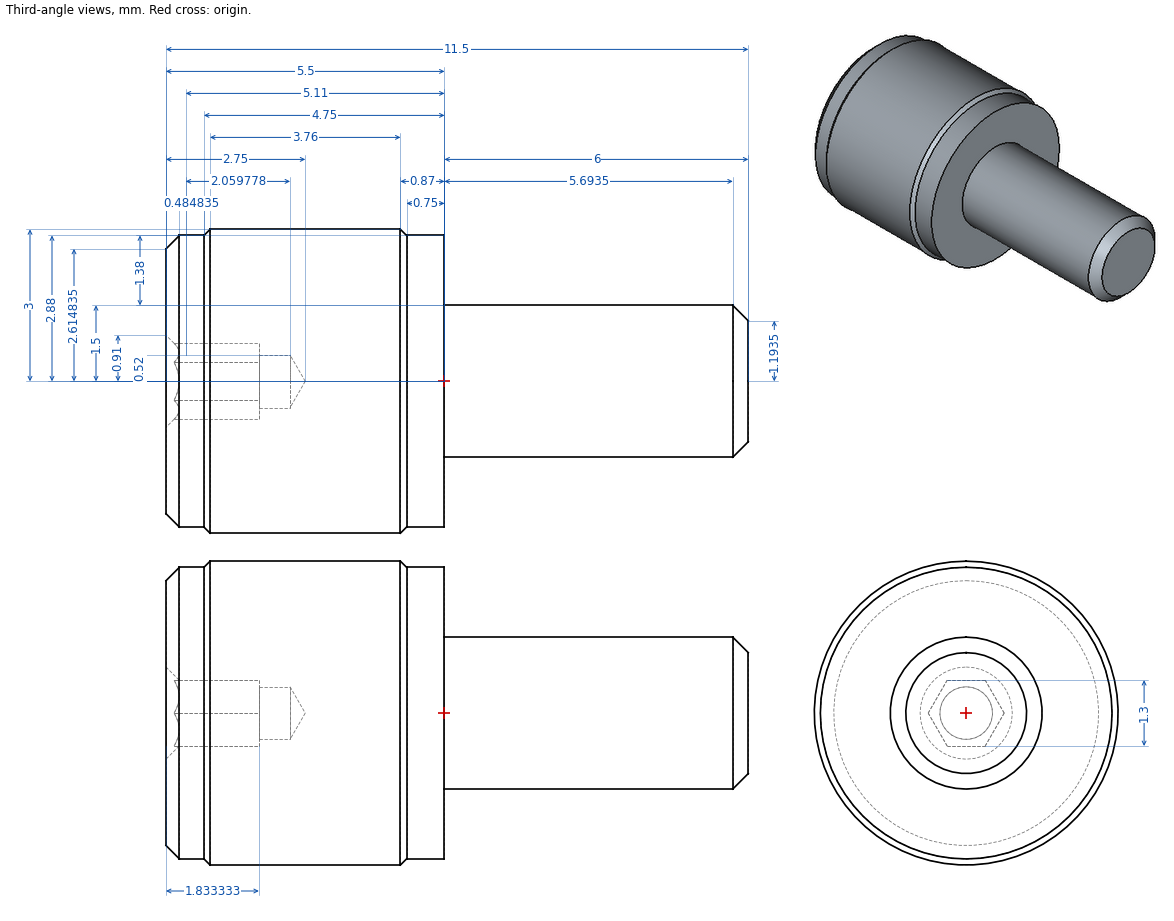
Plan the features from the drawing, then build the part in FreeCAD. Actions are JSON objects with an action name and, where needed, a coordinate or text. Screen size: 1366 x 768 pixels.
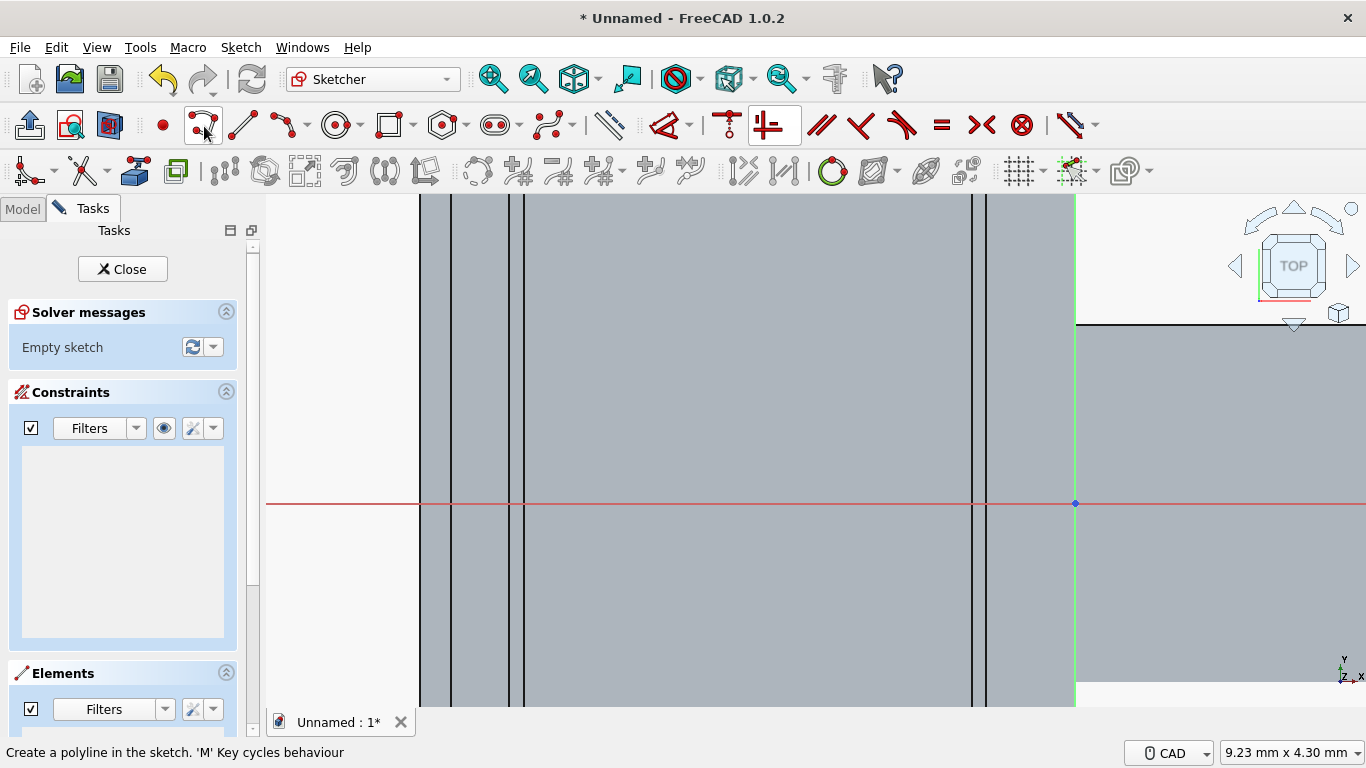
{"action": "left_click", "coordinate": [748, 504]}
{"action": "left_click", "coordinate": [712, 442]}
{"action": "left_click", "coordinate": [466, 442]}
{"action": "left_click", "coordinate": [420, 396]}
{"action": "left_click", "coordinate": [420, 495]}
{"action": "left_click", "coordinate": [748, 504]}
{"action": "key", "text": "Escape"}
{"action": "key", "text": "Escape"}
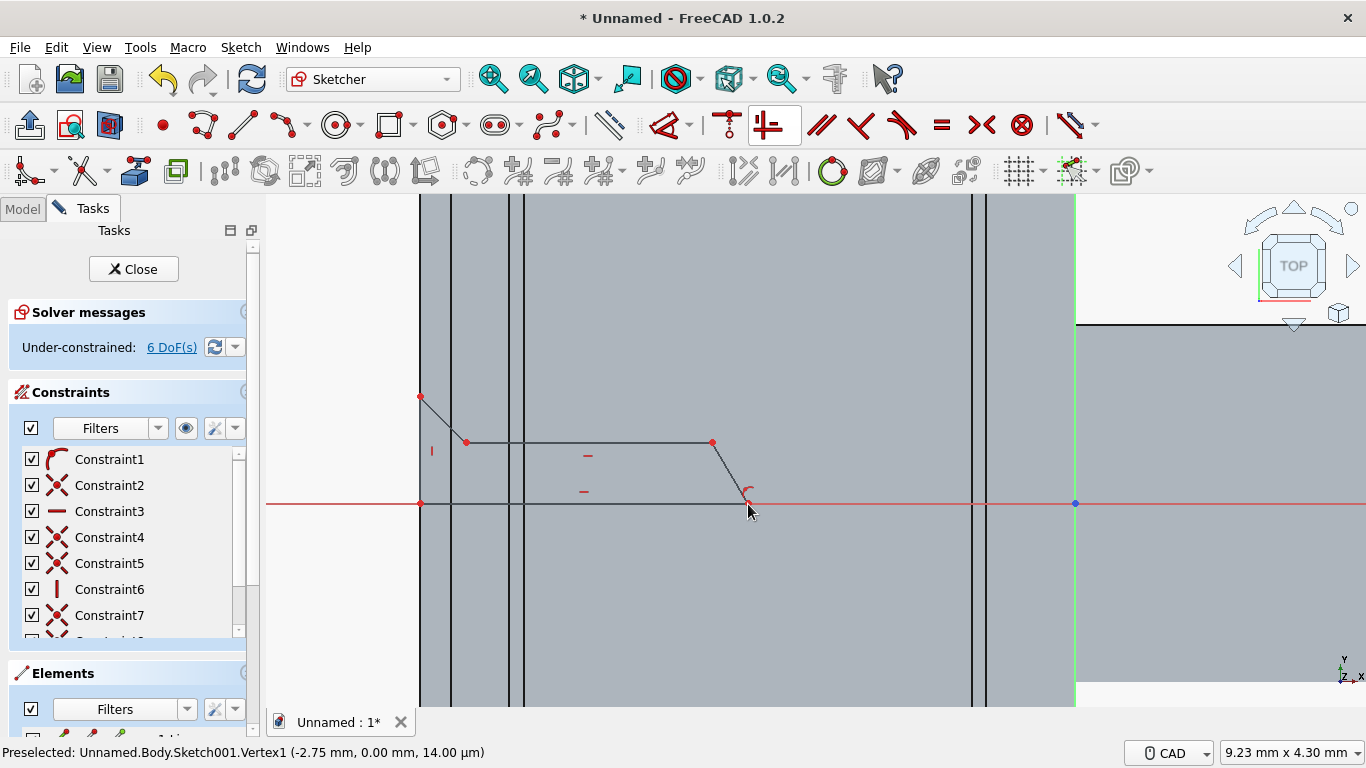
{"action": "key", "text": "d"}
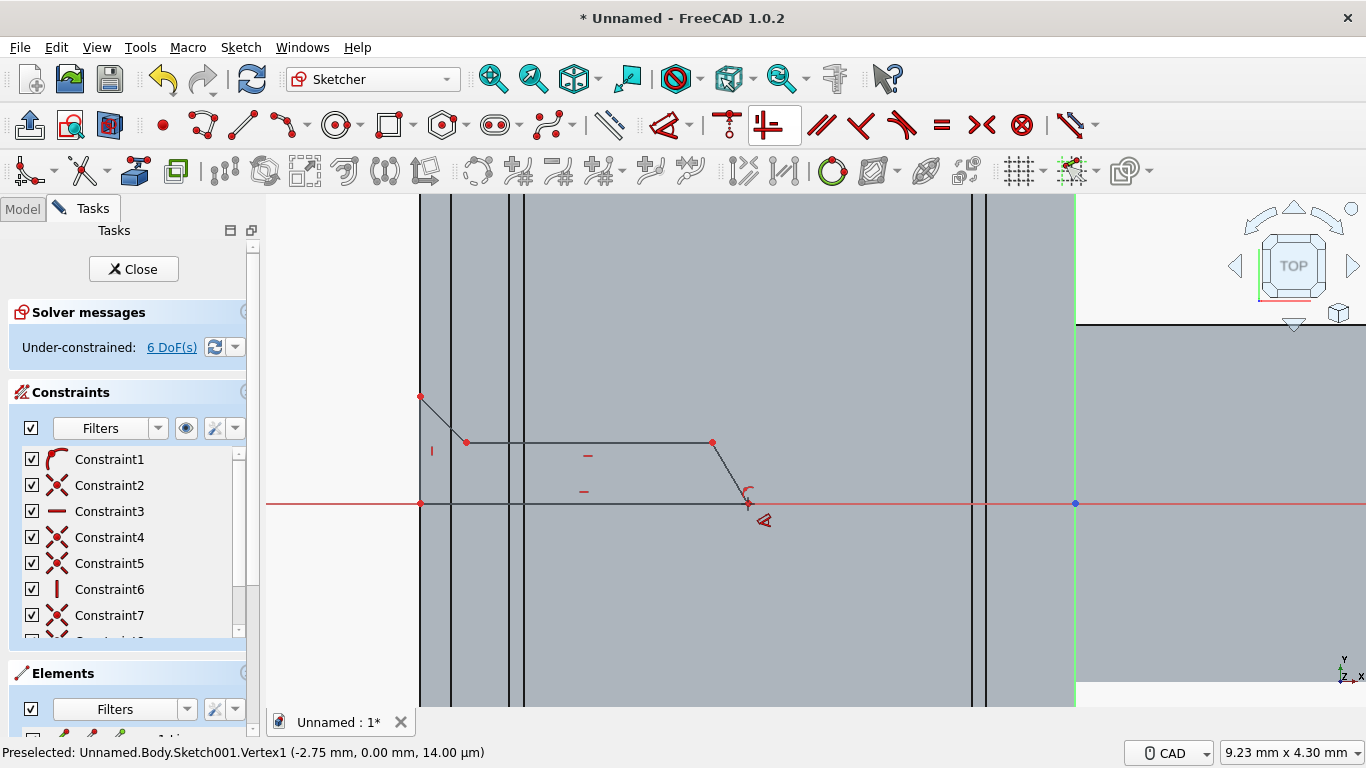
{"action": "left_click", "coordinate": [420, 429]}
{"action": "left_click", "coordinate": [386, 450]}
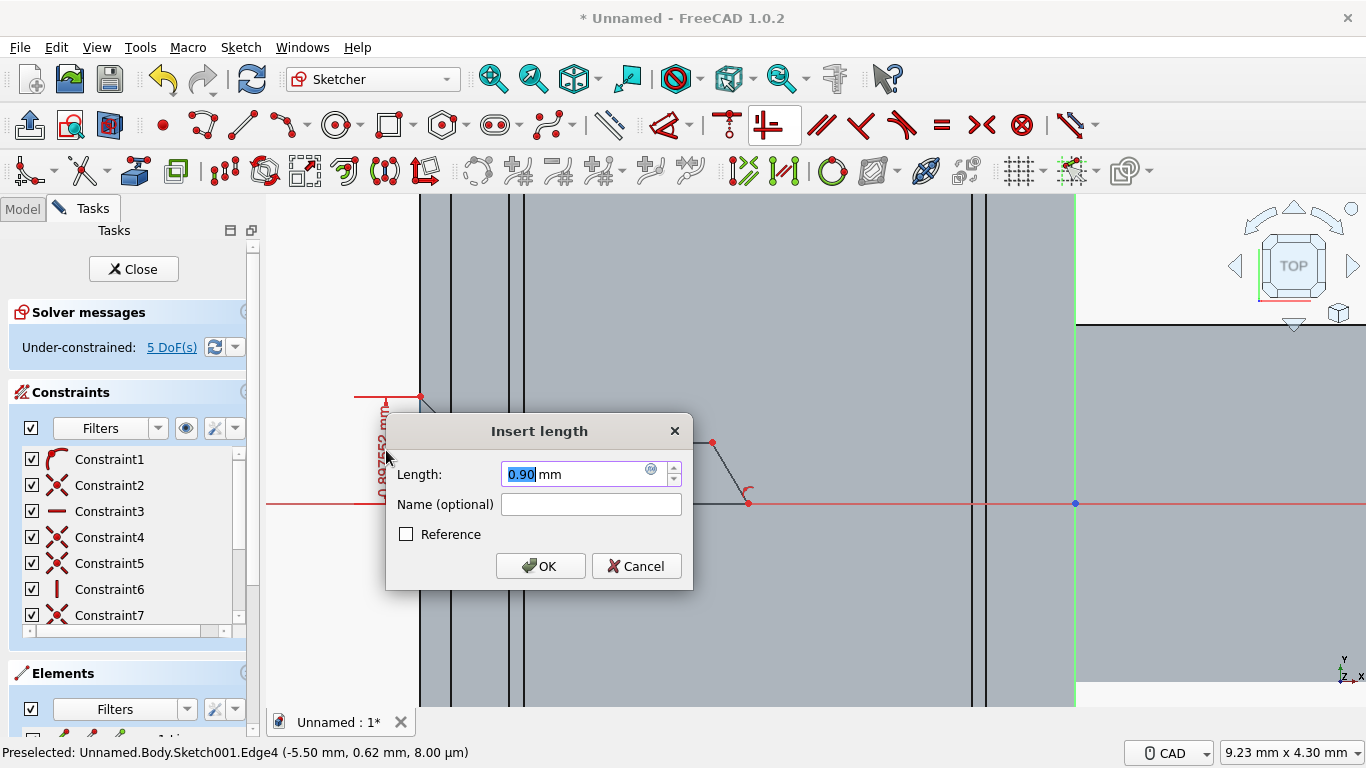
{"action": "type", "text": "0.91"}
{"action": "key", "text": "Return"}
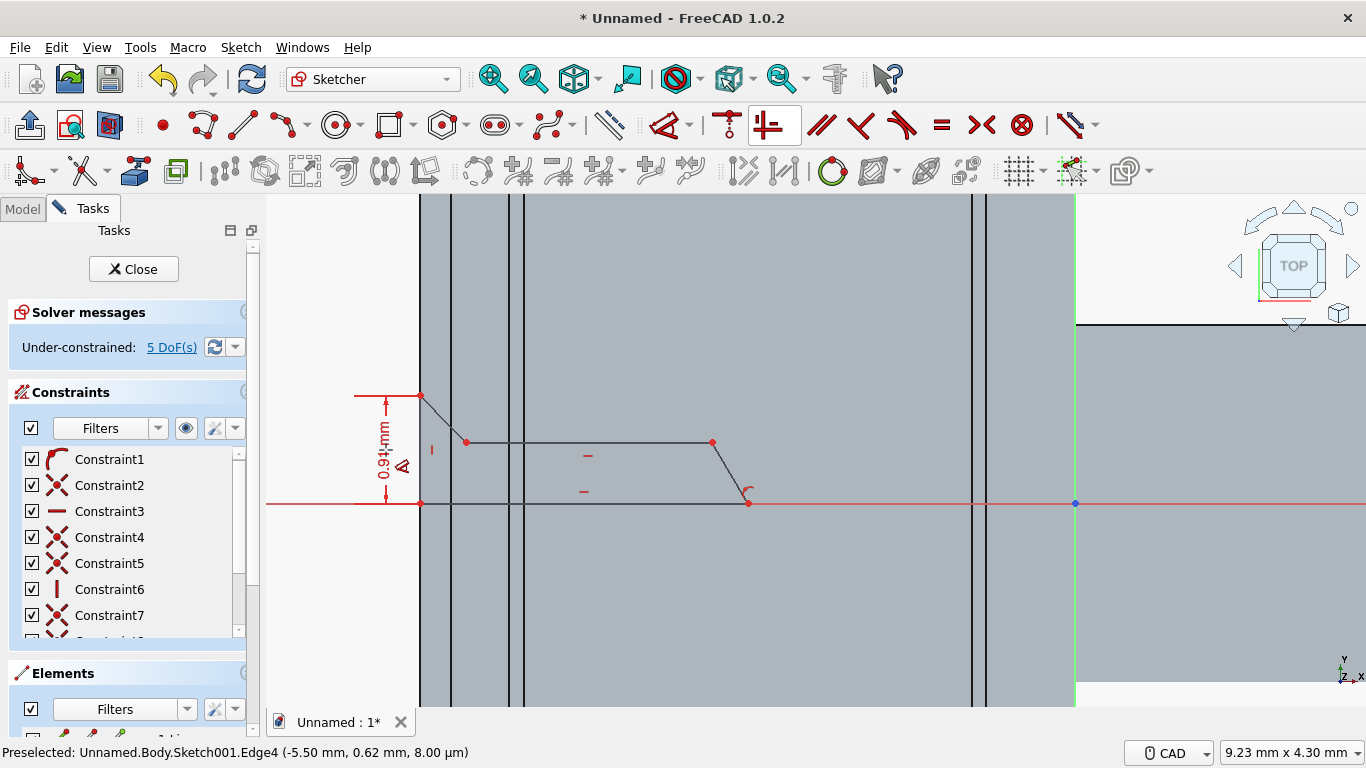
{"action": "left_click", "coordinate": [518, 504]}
{"action": "left_click", "coordinate": [584, 538]}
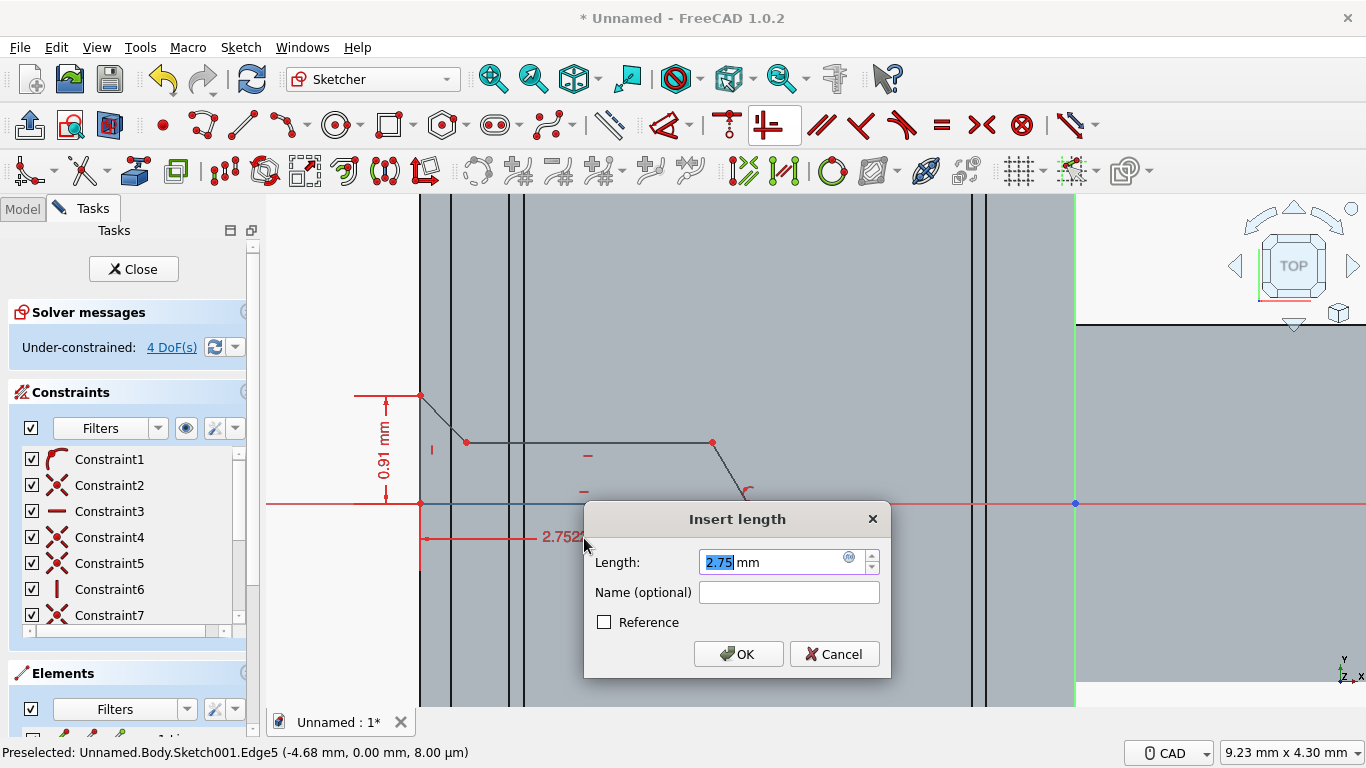
{"action": "type", "text": "2.75"}
{"action": "key", "text": "Return"}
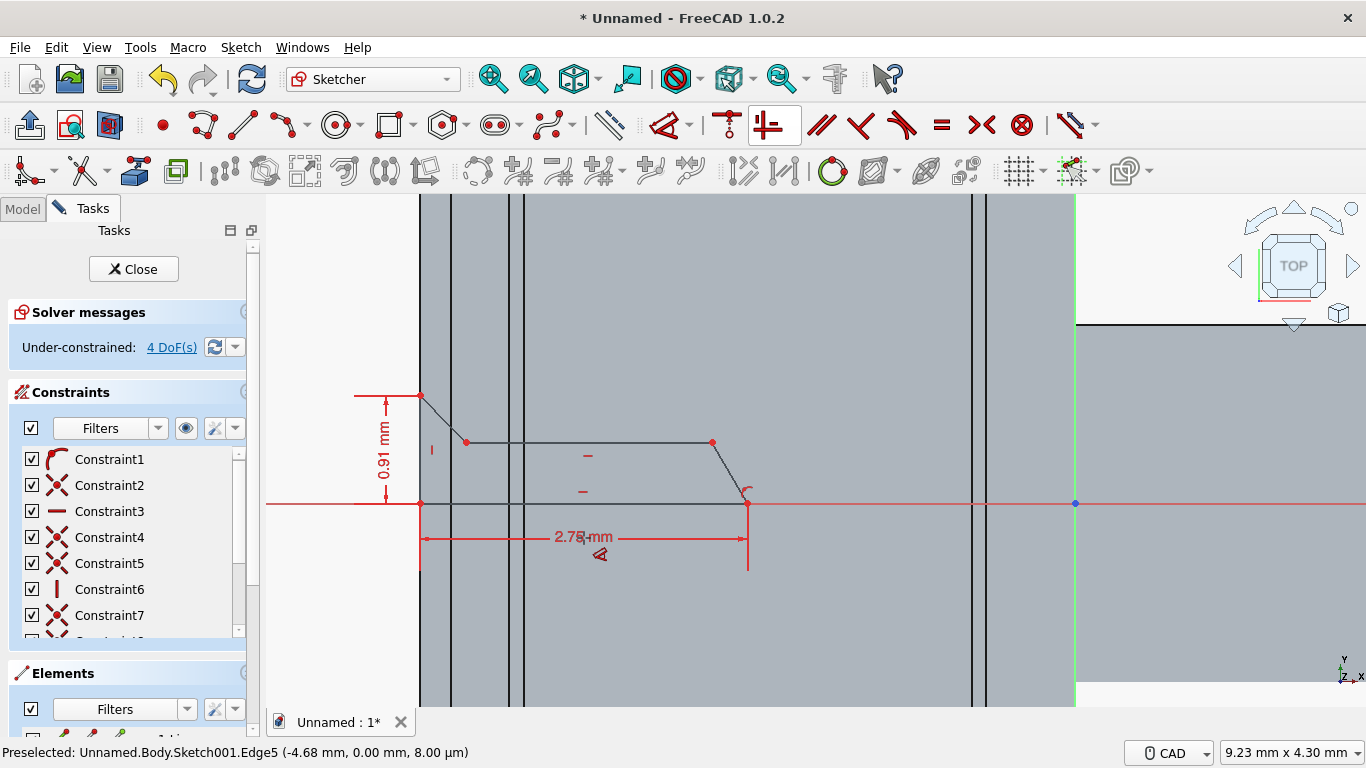
{"action": "left_click", "coordinate": [420, 396]}
{"action": "left_click", "coordinate": [748, 538]}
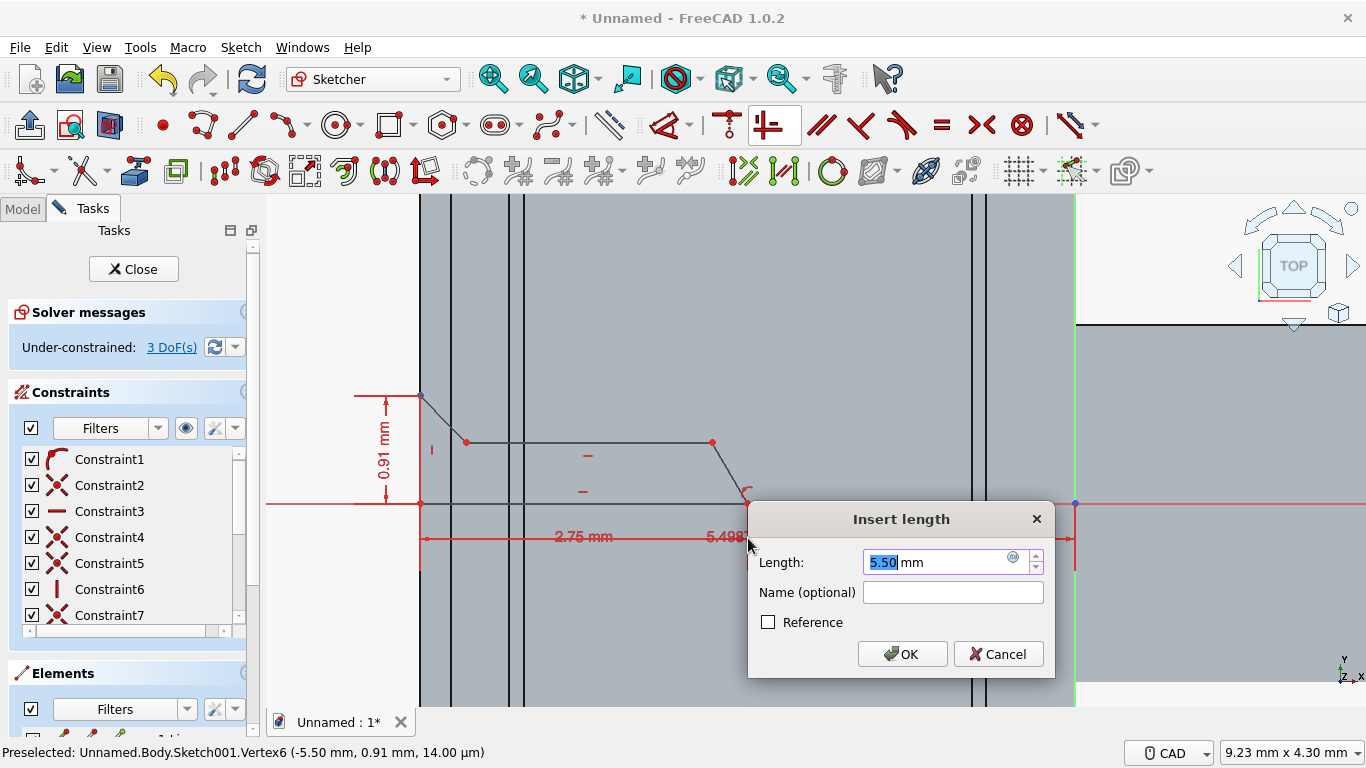
{"action": "type", "text": "5.5"}
{"action": "key", "text": "Return"}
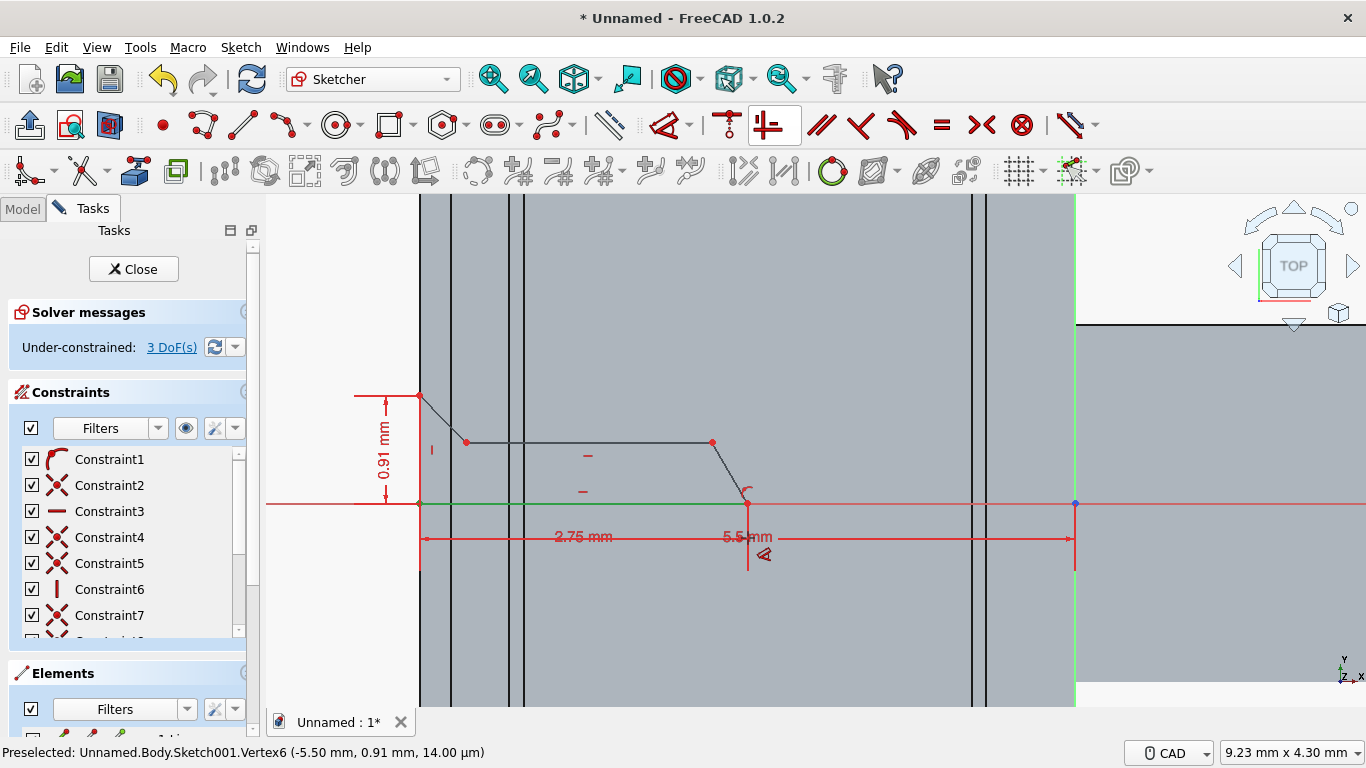
{"action": "left_click", "coordinate": [712, 443]}
{"action": "left_click", "coordinate": [1109, 473]}